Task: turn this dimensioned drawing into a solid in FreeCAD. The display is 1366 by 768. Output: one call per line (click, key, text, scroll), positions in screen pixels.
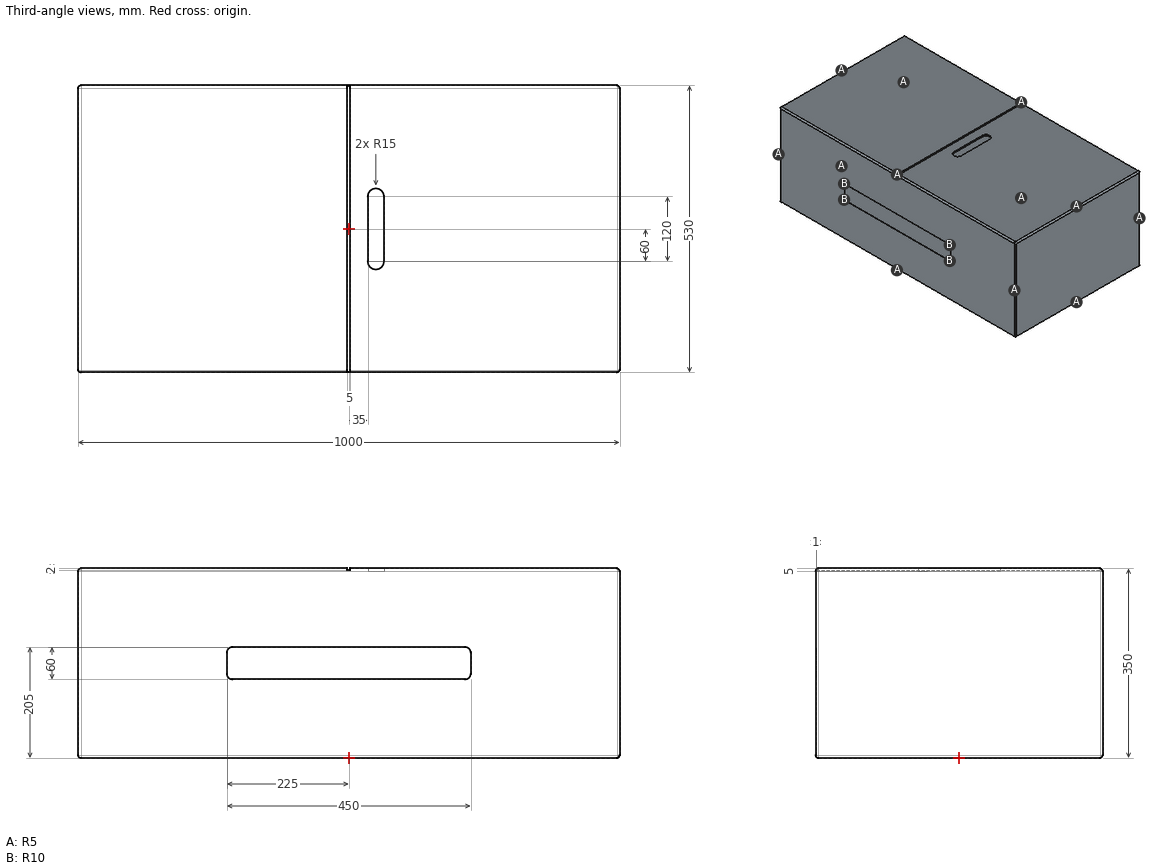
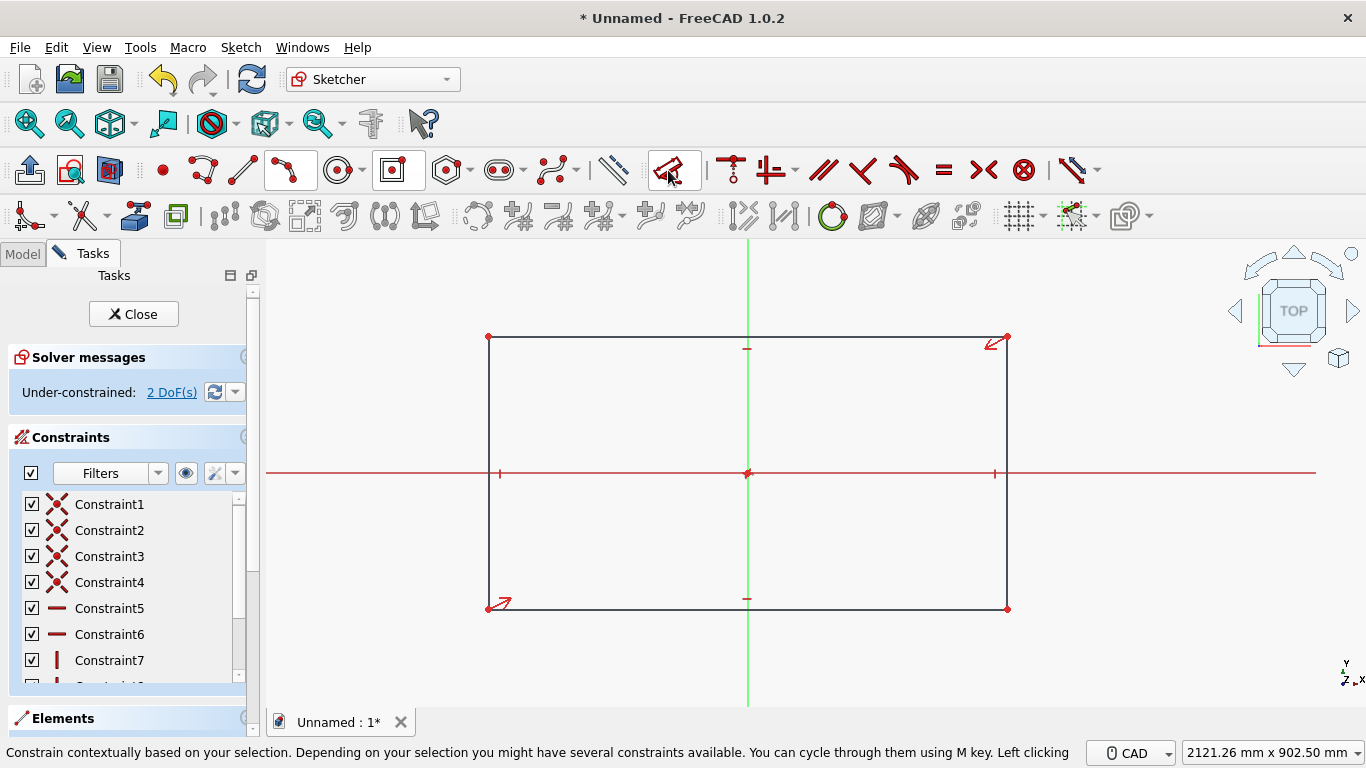
click(1007, 528)
click(1041, 411)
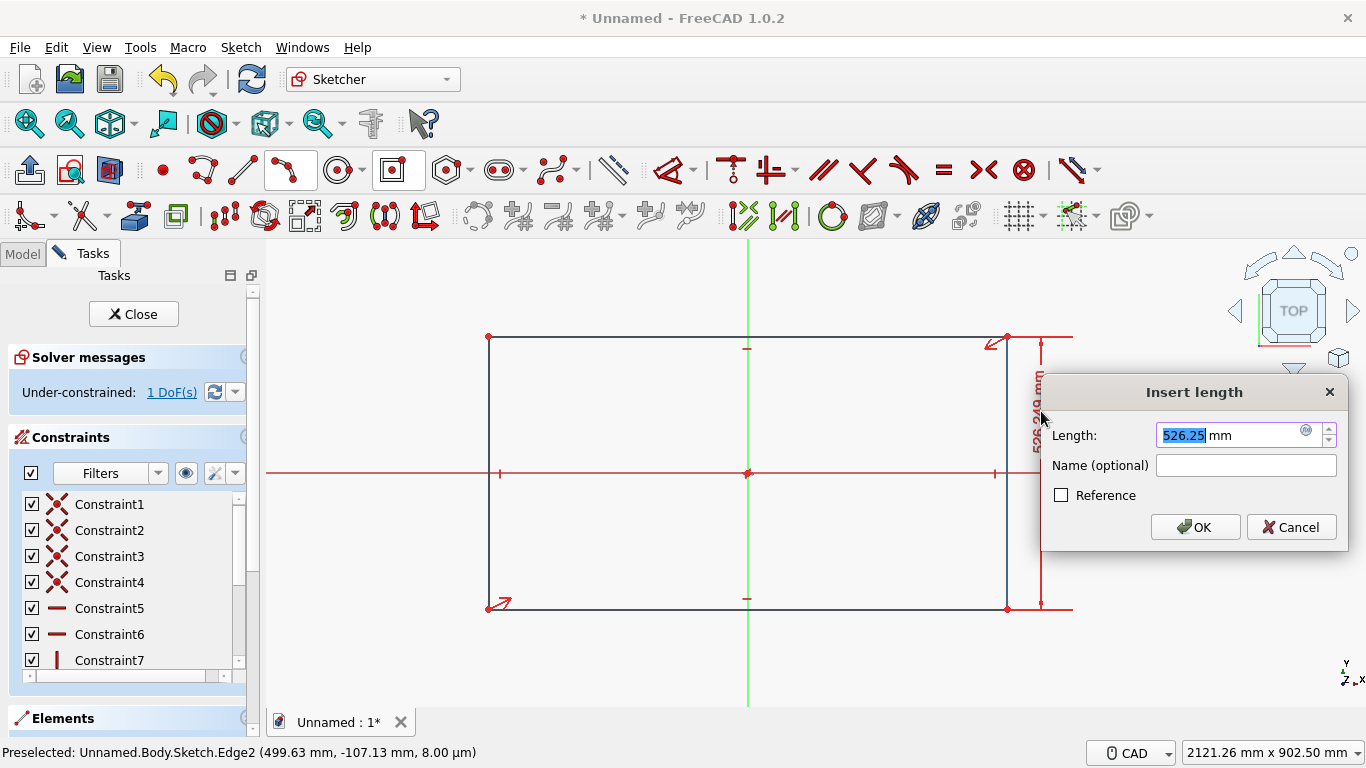
text(530)
key(Return)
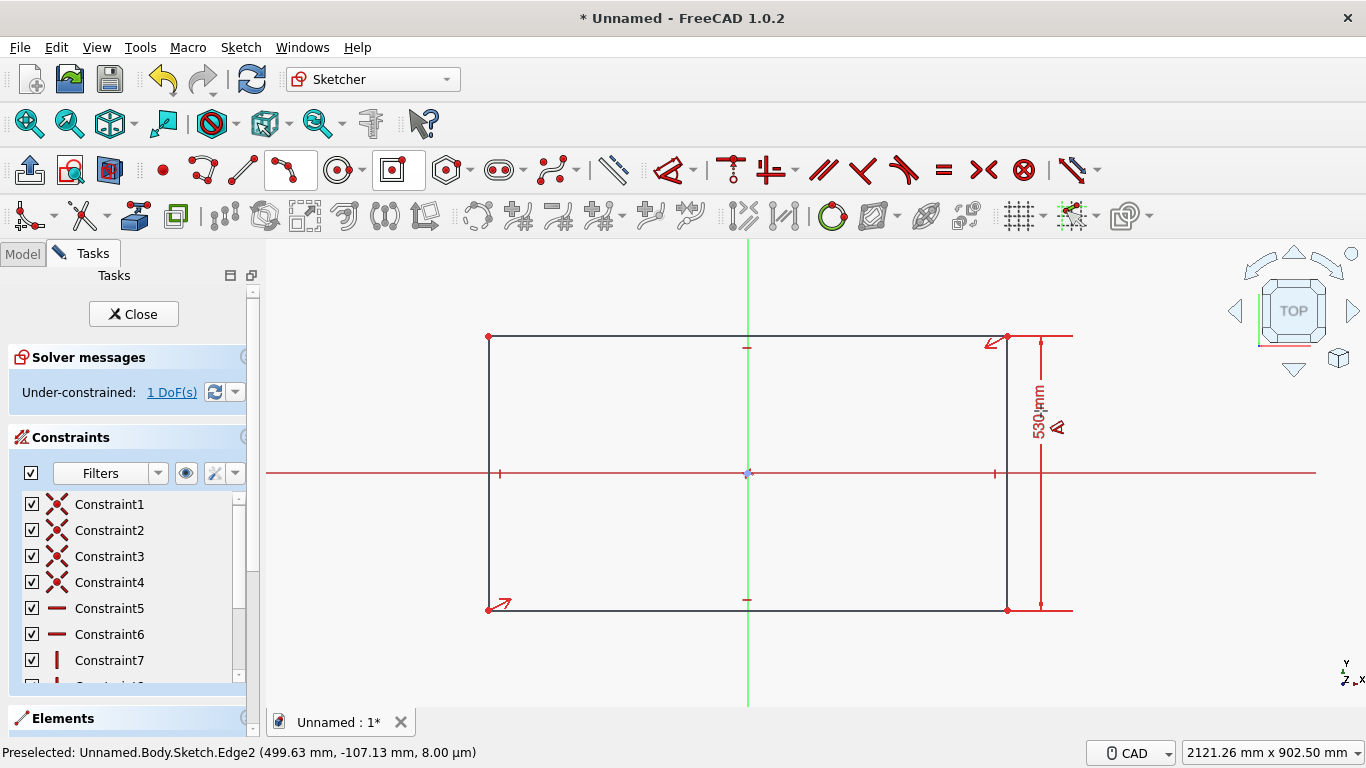
click(644, 611)
click(629, 645)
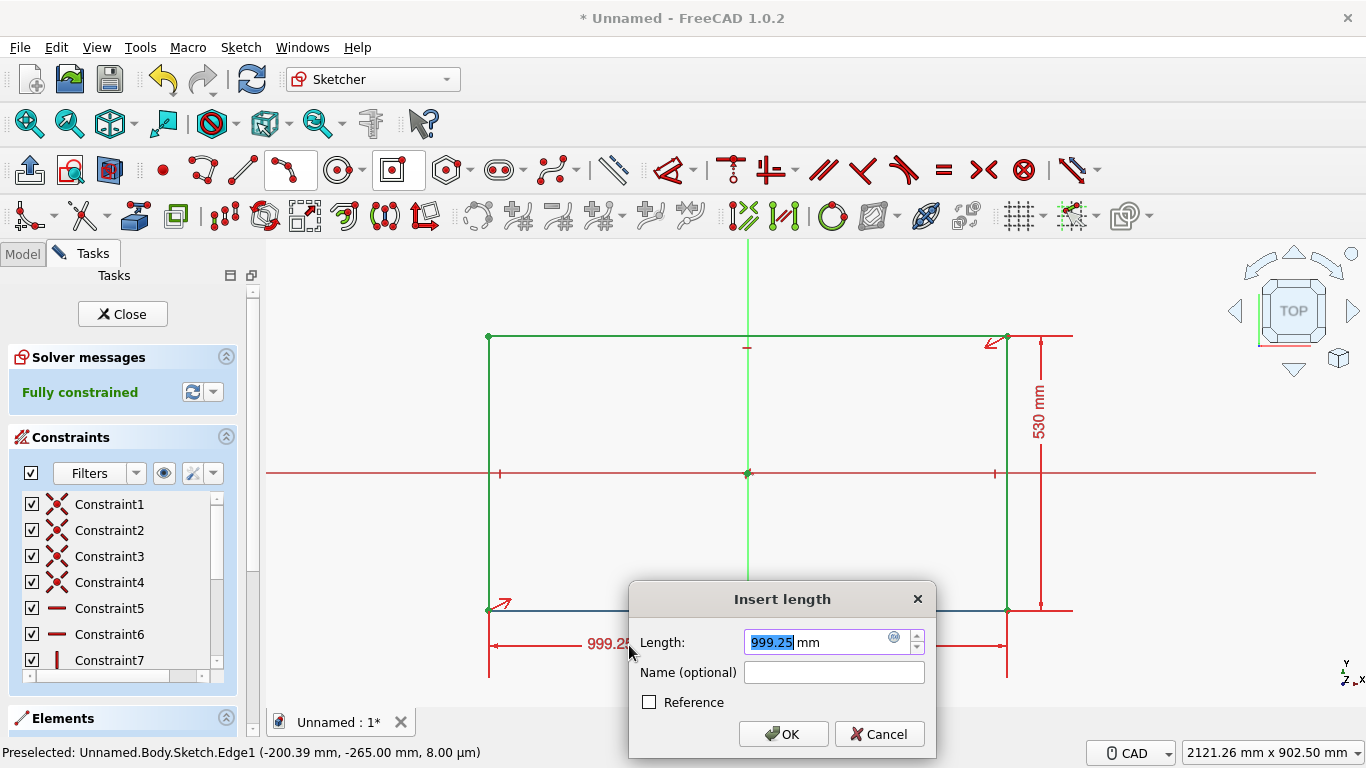
text(1000)
key(Return)
key(Escape)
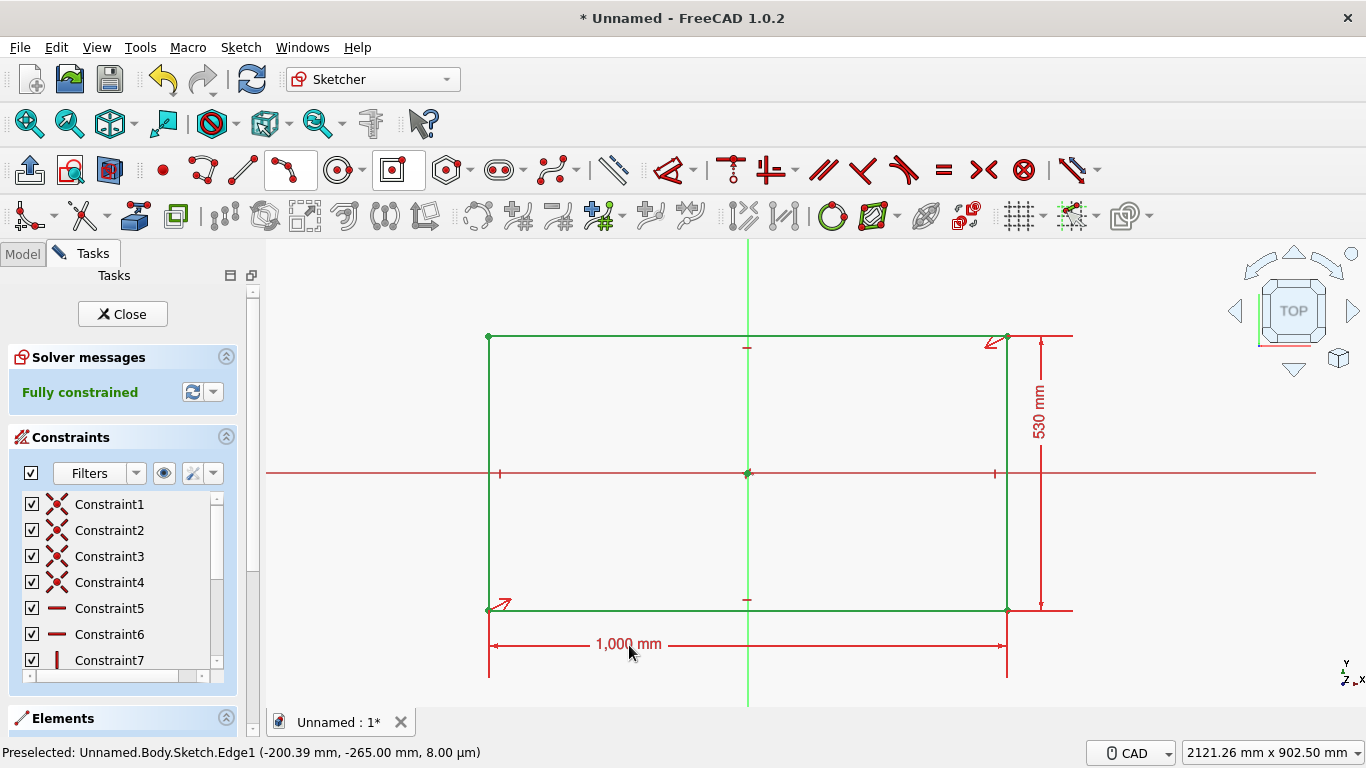
click(123, 314)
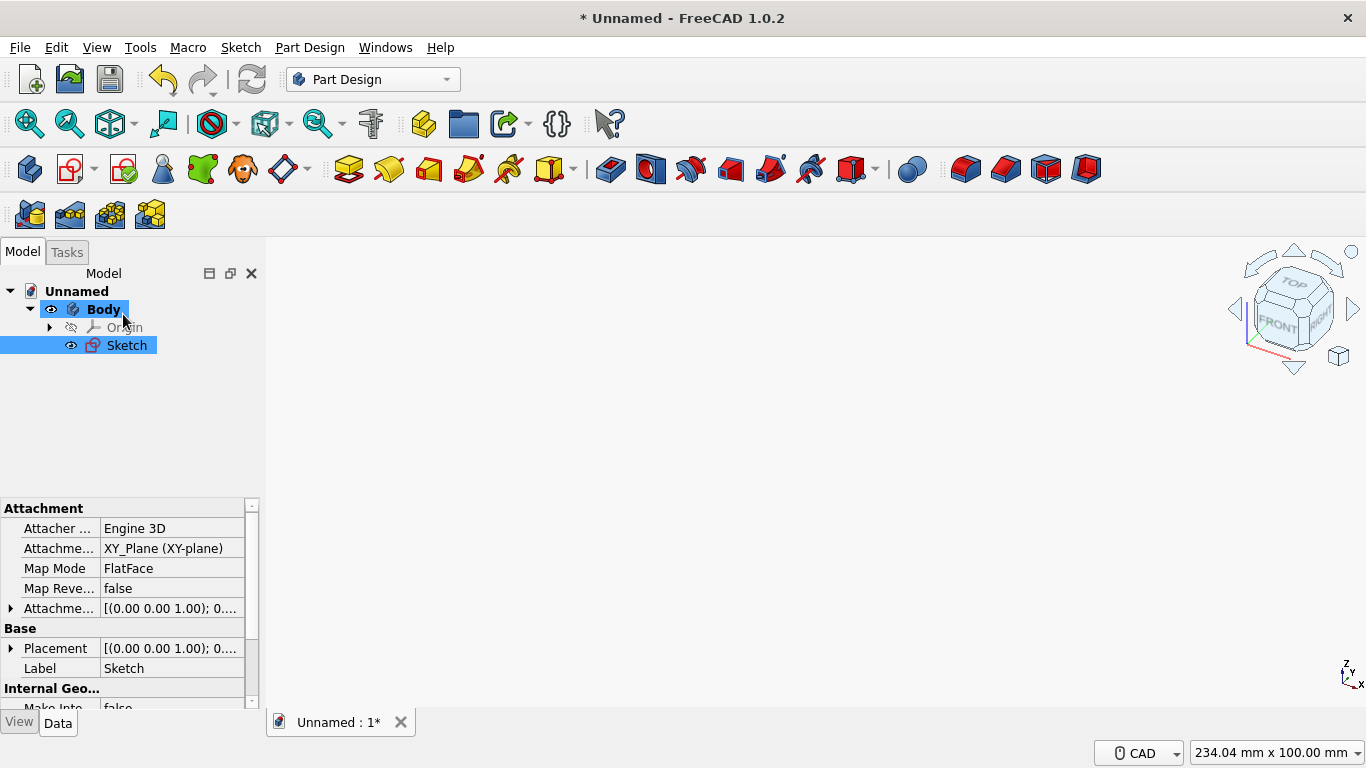
click(350, 170)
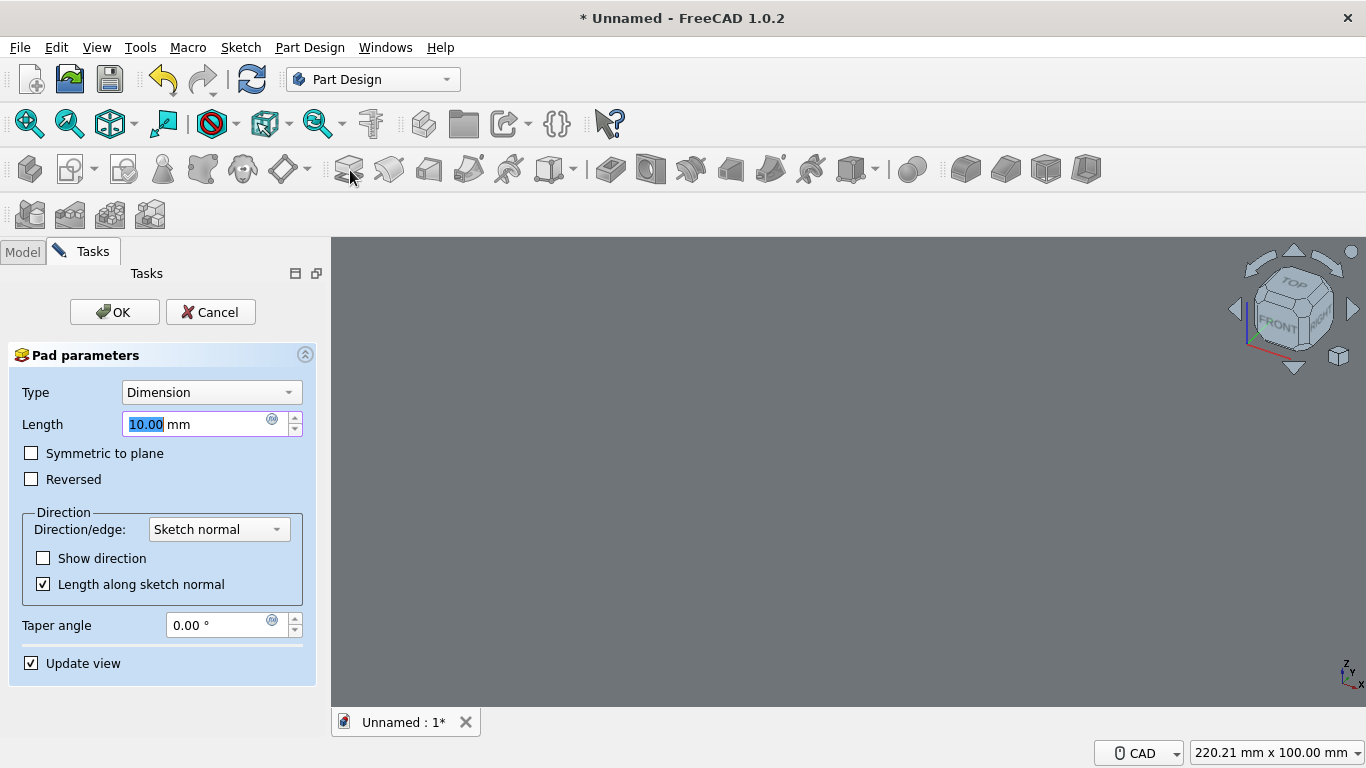
text(350)
key(Tab)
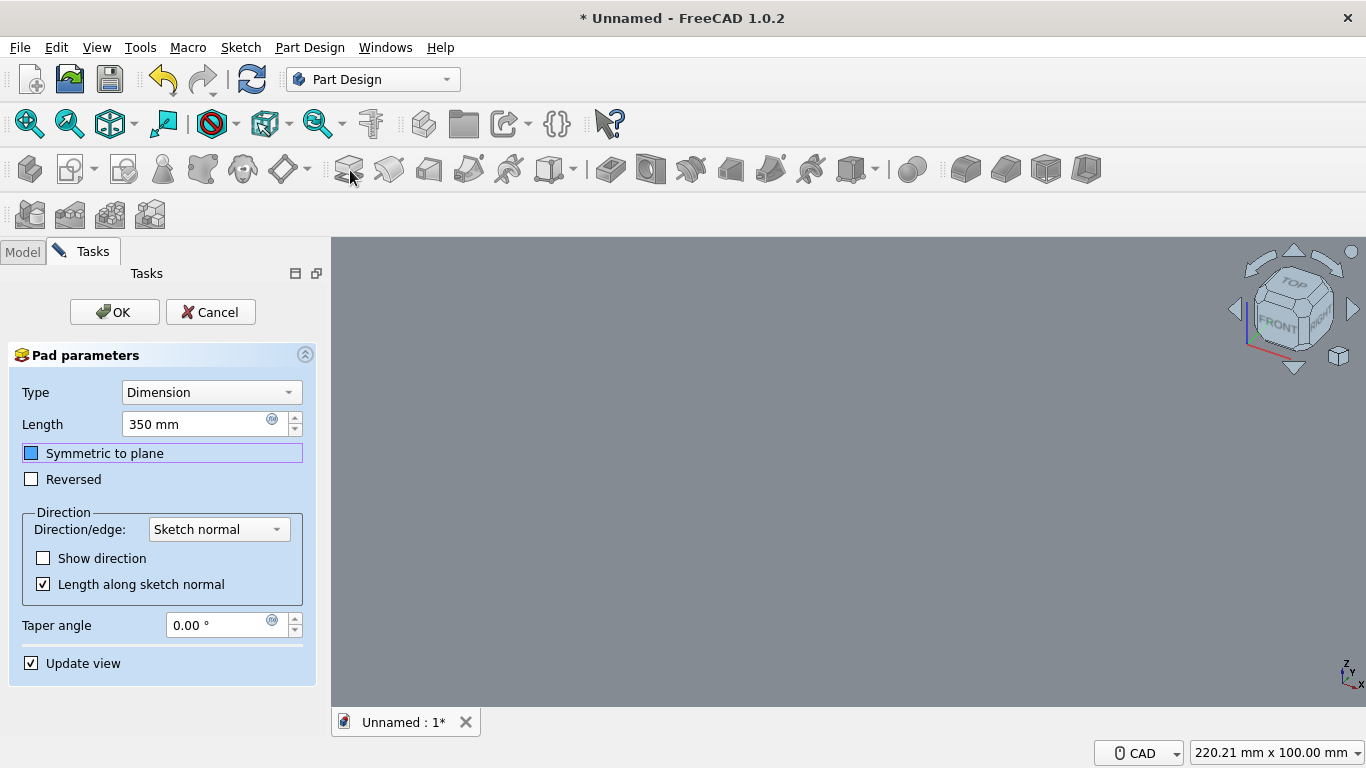
click(115, 312)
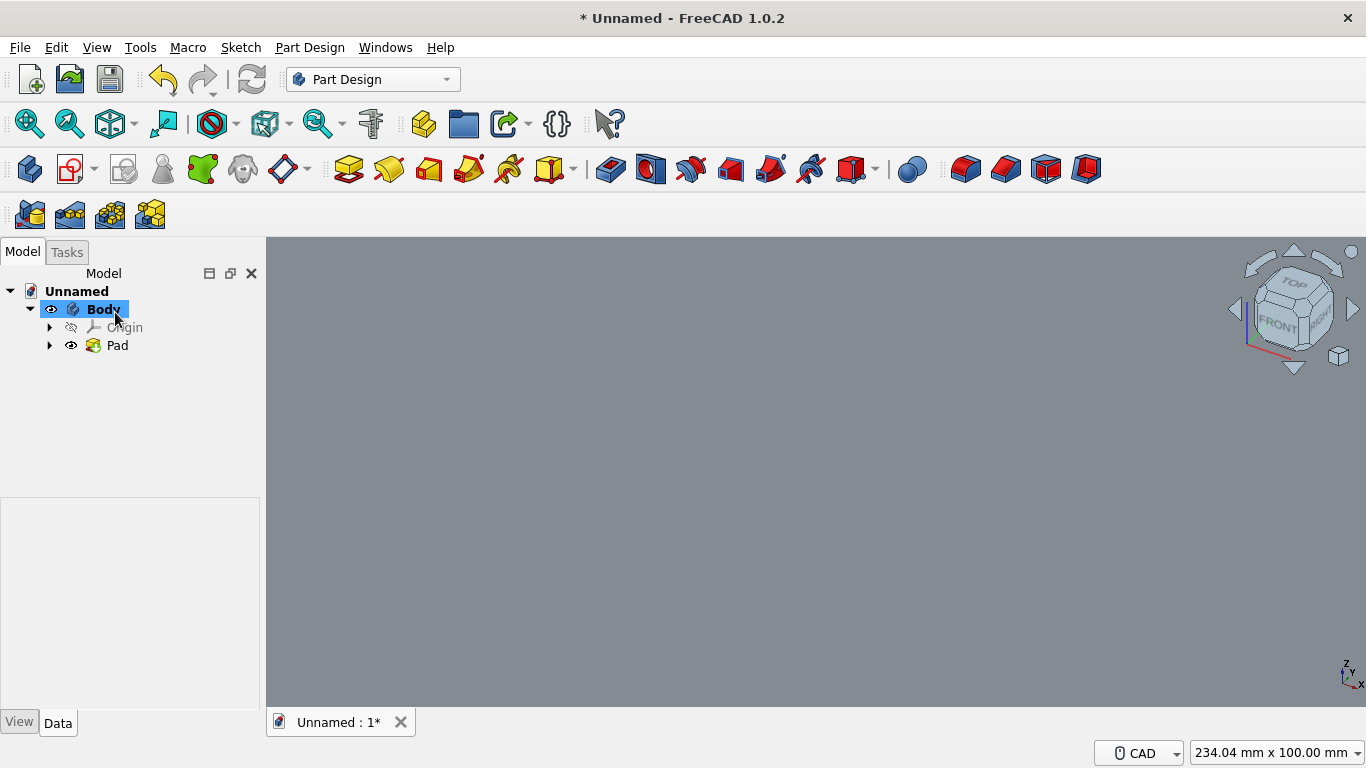
click(30, 124)